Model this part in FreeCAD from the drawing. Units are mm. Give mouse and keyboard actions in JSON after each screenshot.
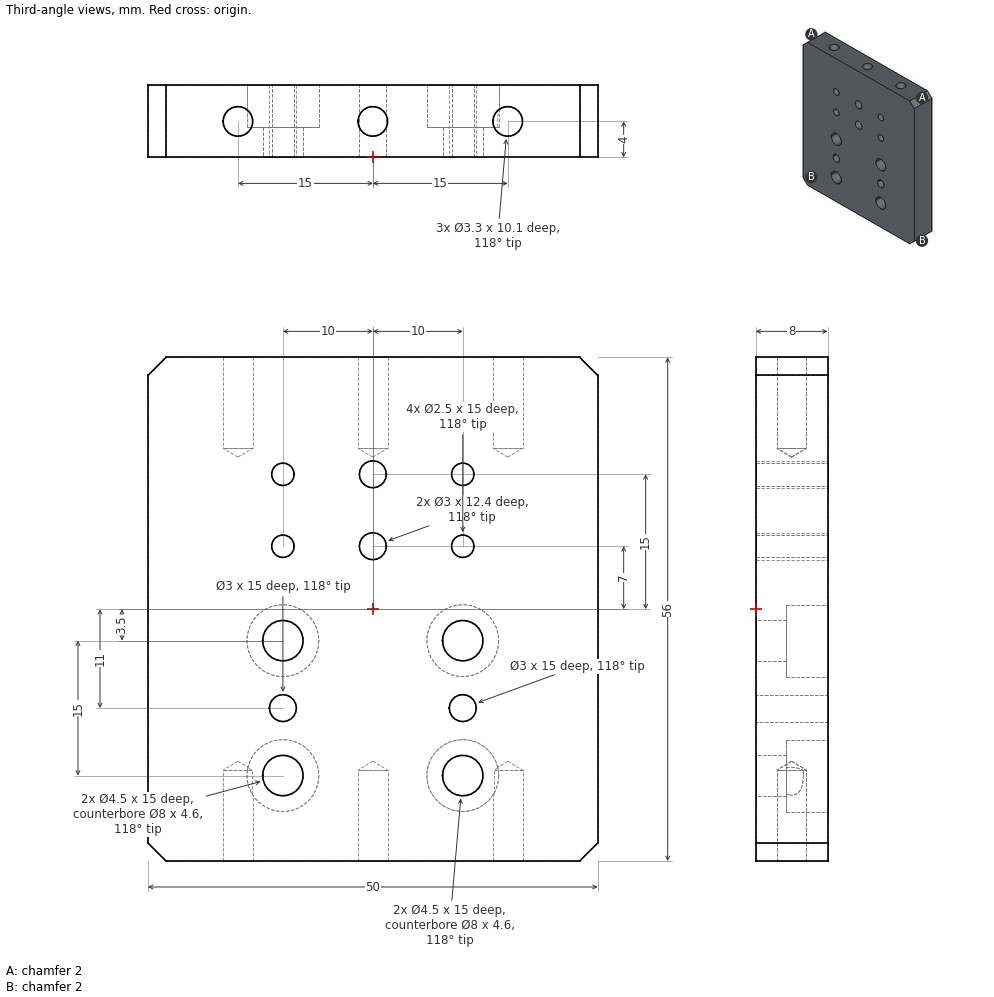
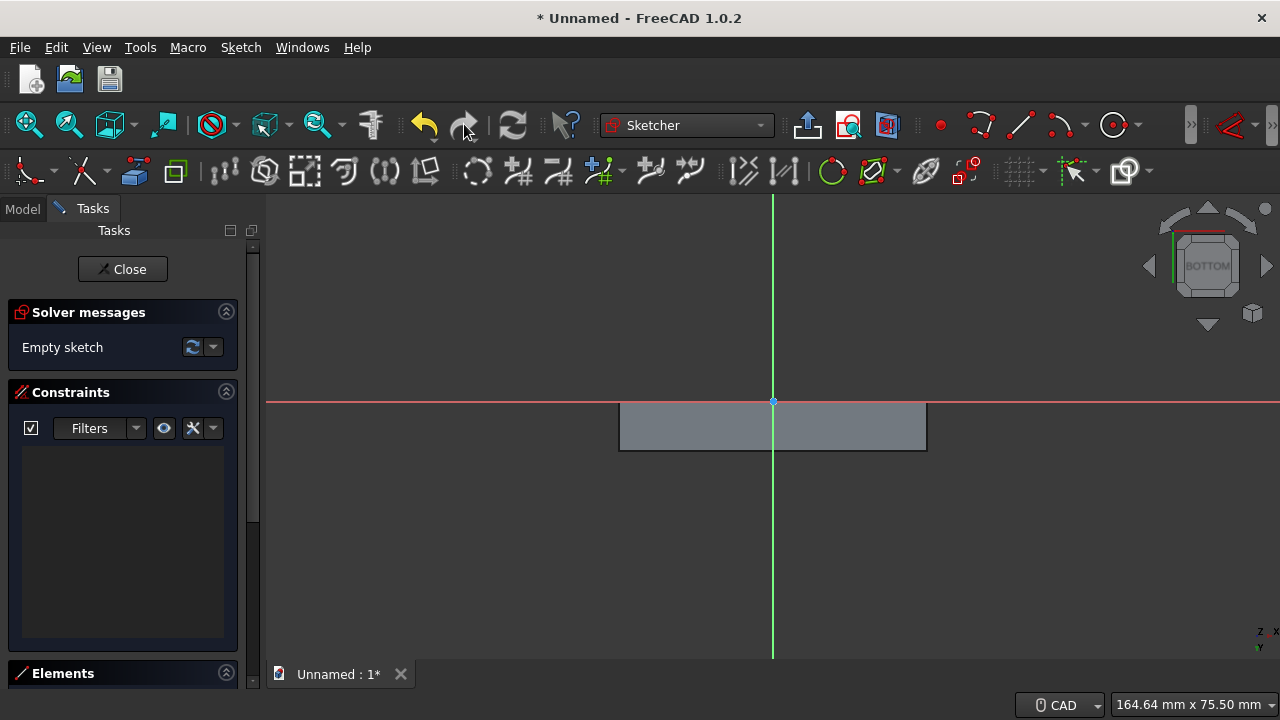
{"action": "scroll", "coordinate": [813, 415], "scroll_direction": "up", "scroll_amount": 5}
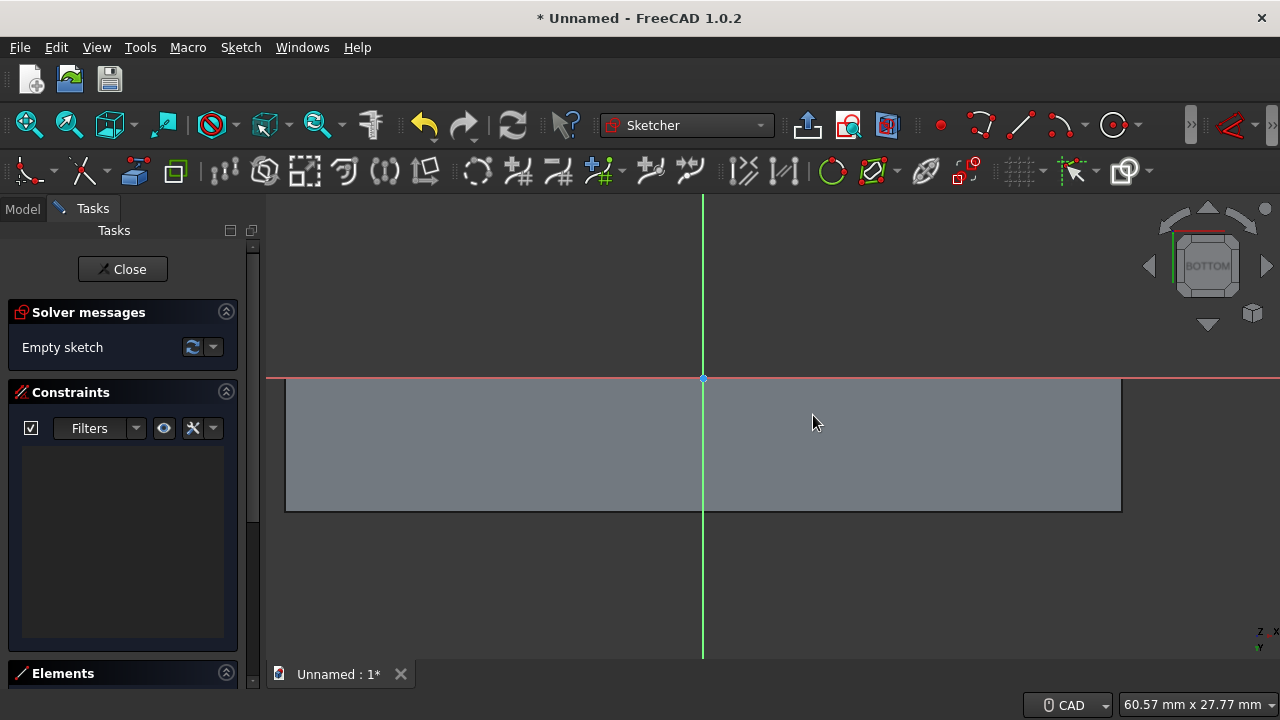
{"action": "left_click", "coordinate": [1114, 126]}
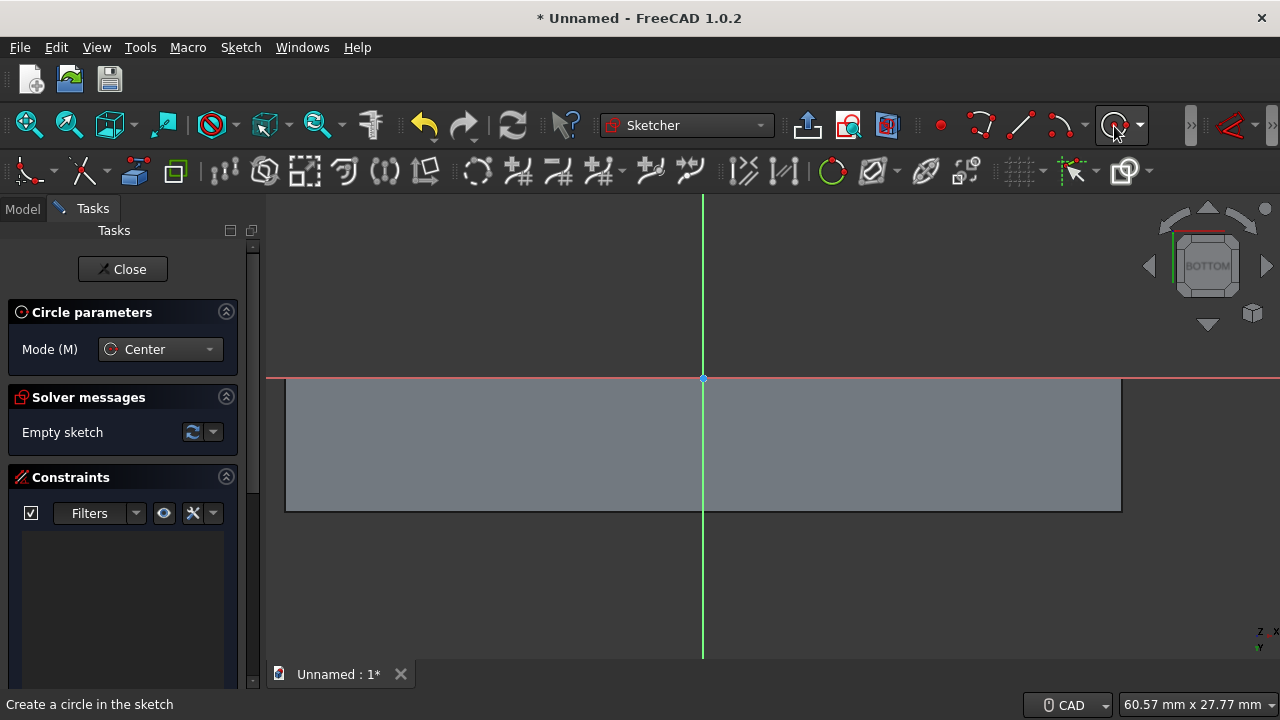
{"action": "left_click", "coordinate": [954, 445]}
{"action": "mouse_move", "coordinate": [974, 426]}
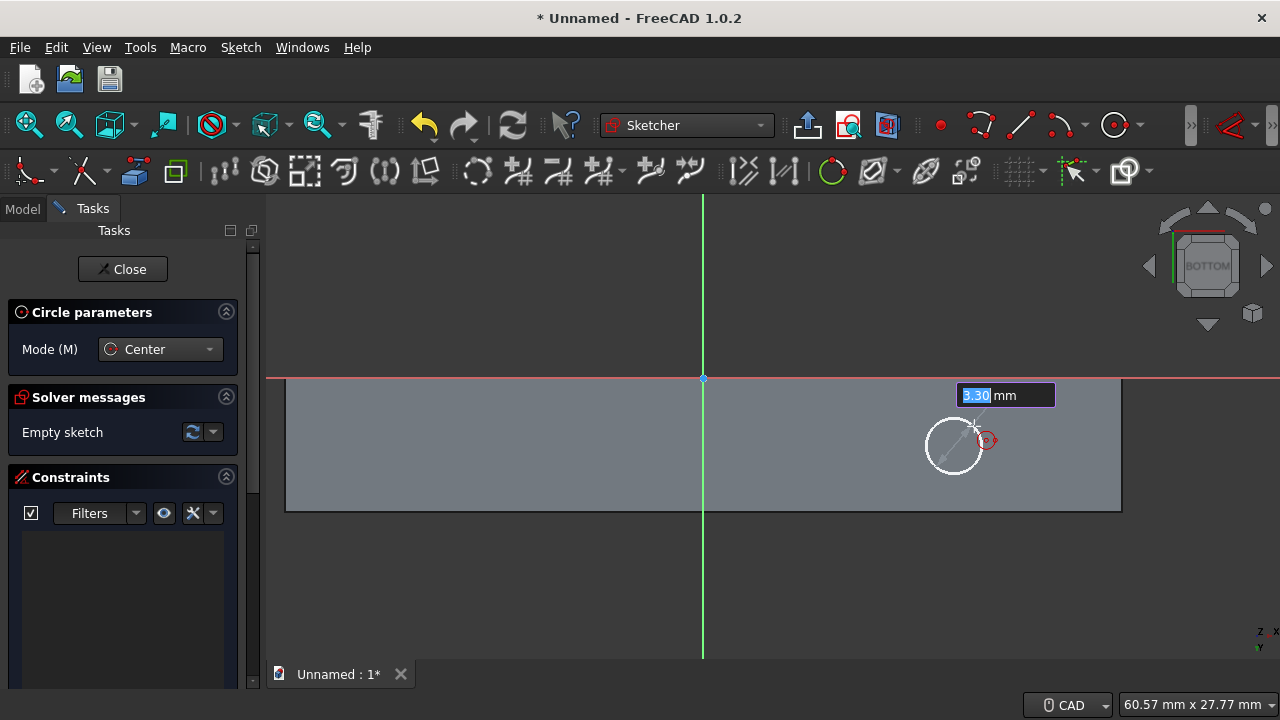
{"action": "type", "text": "3.3"}
{"action": "key", "text": "Return"}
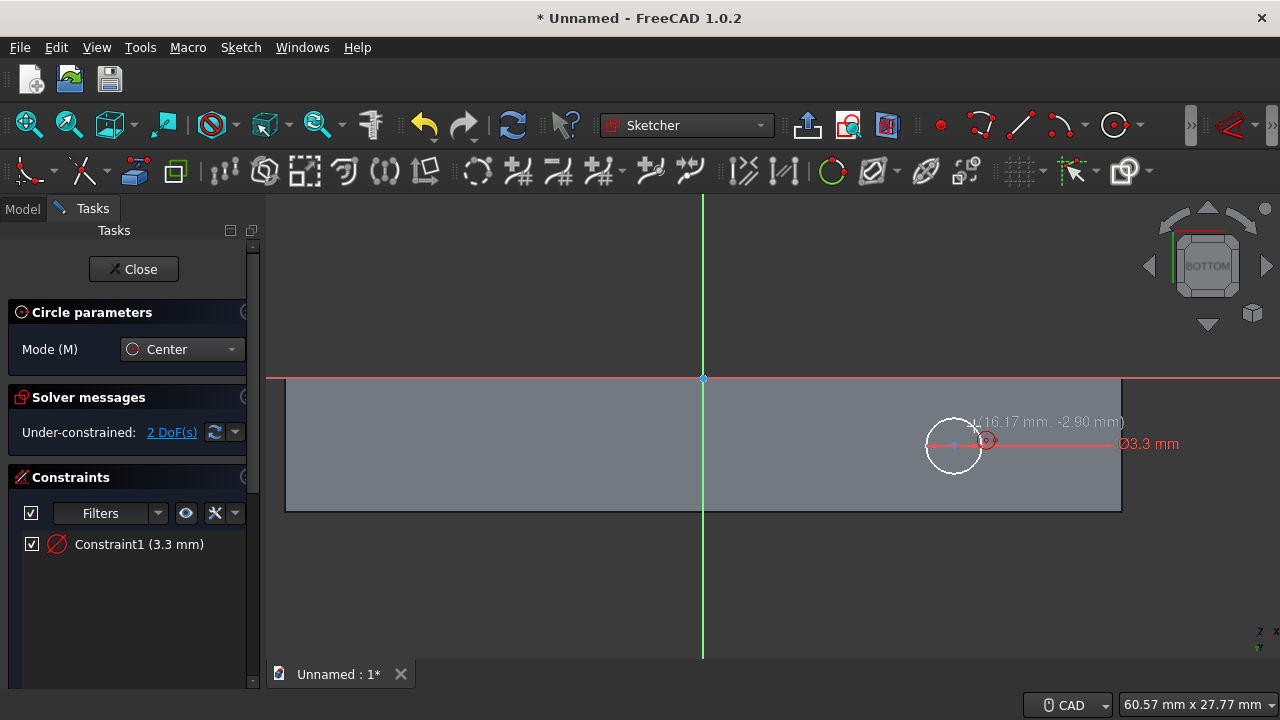
{"action": "left_click", "coordinate": [703, 445]}
{"action": "mouse_move", "coordinate": [723, 426]}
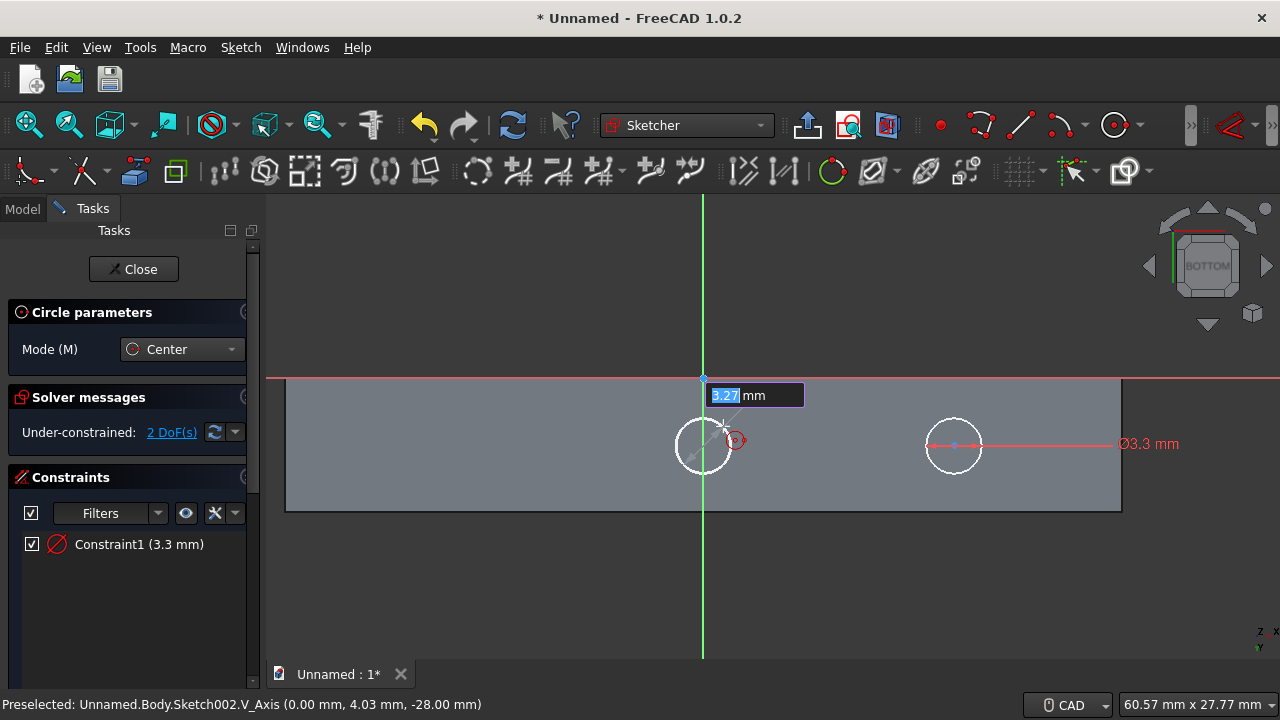
{"action": "type", "text": "3.3"}
{"action": "key", "text": "Return"}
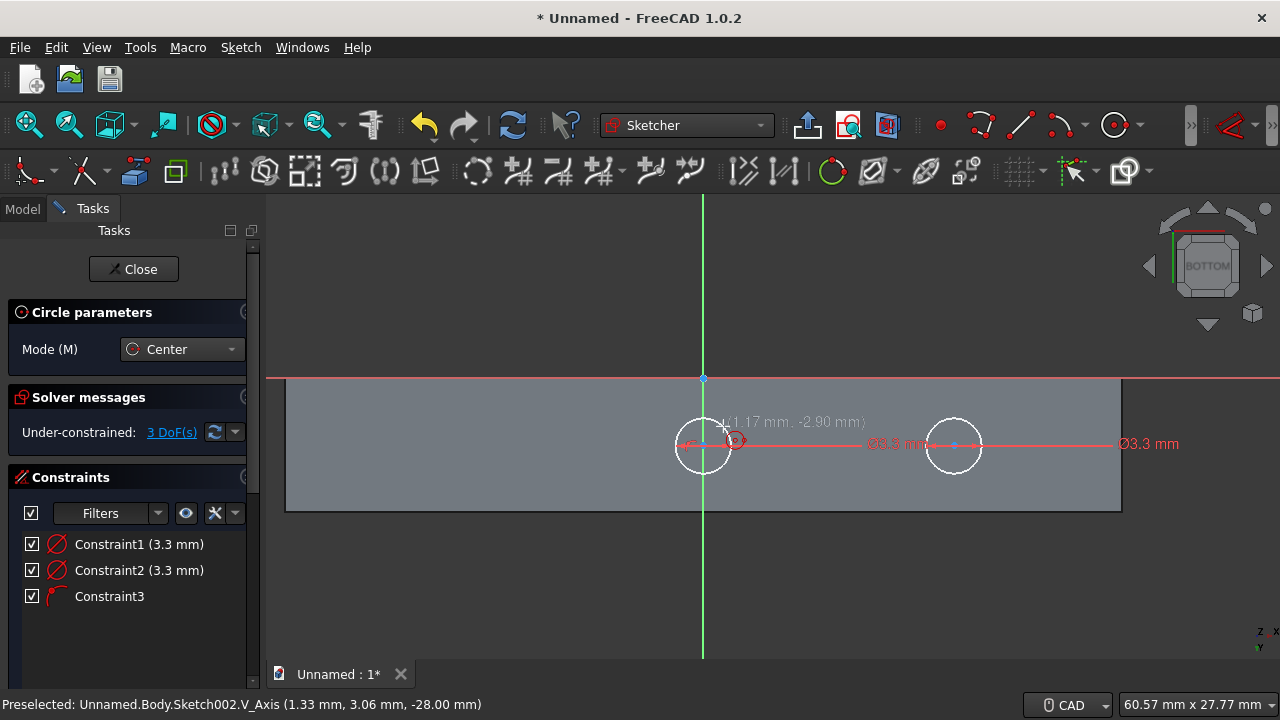
{"action": "left_click", "coordinate": [452, 445]}
{"action": "mouse_move", "coordinate": [472, 426]}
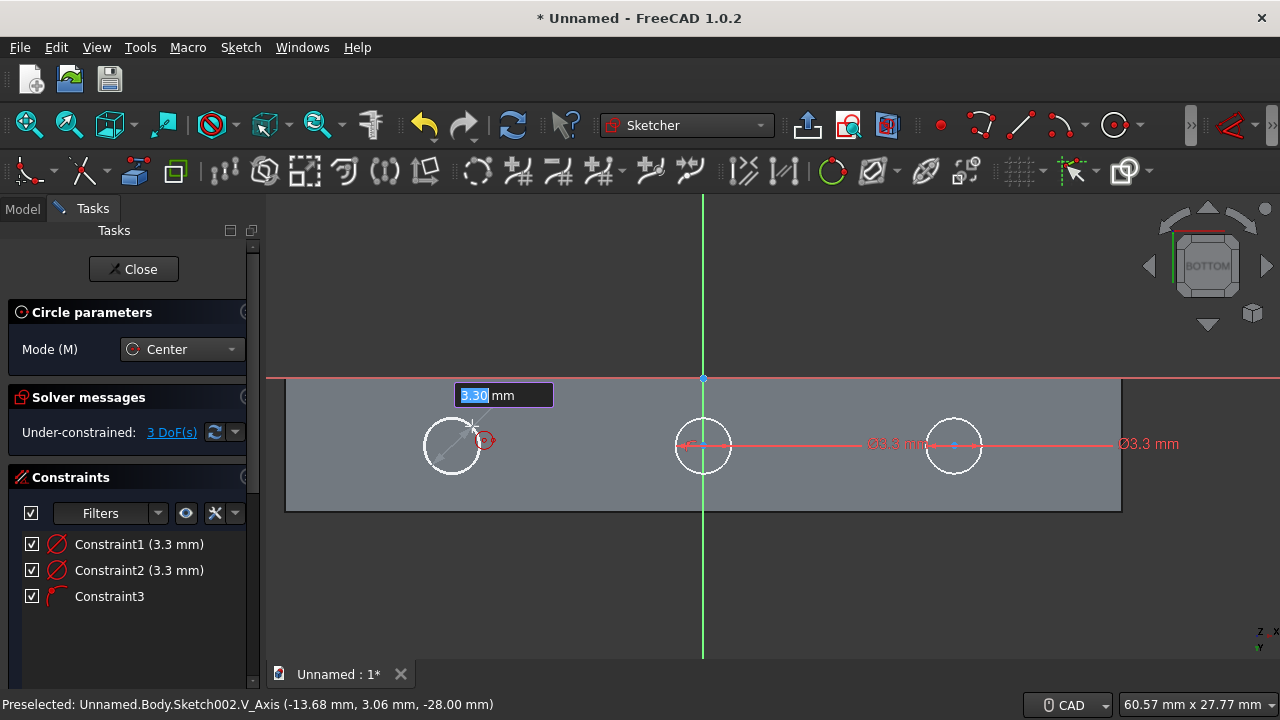
{"action": "type", "text": "3.3"}
{"action": "key", "text": "Return"}
{"action": "key", "text": "Escape"}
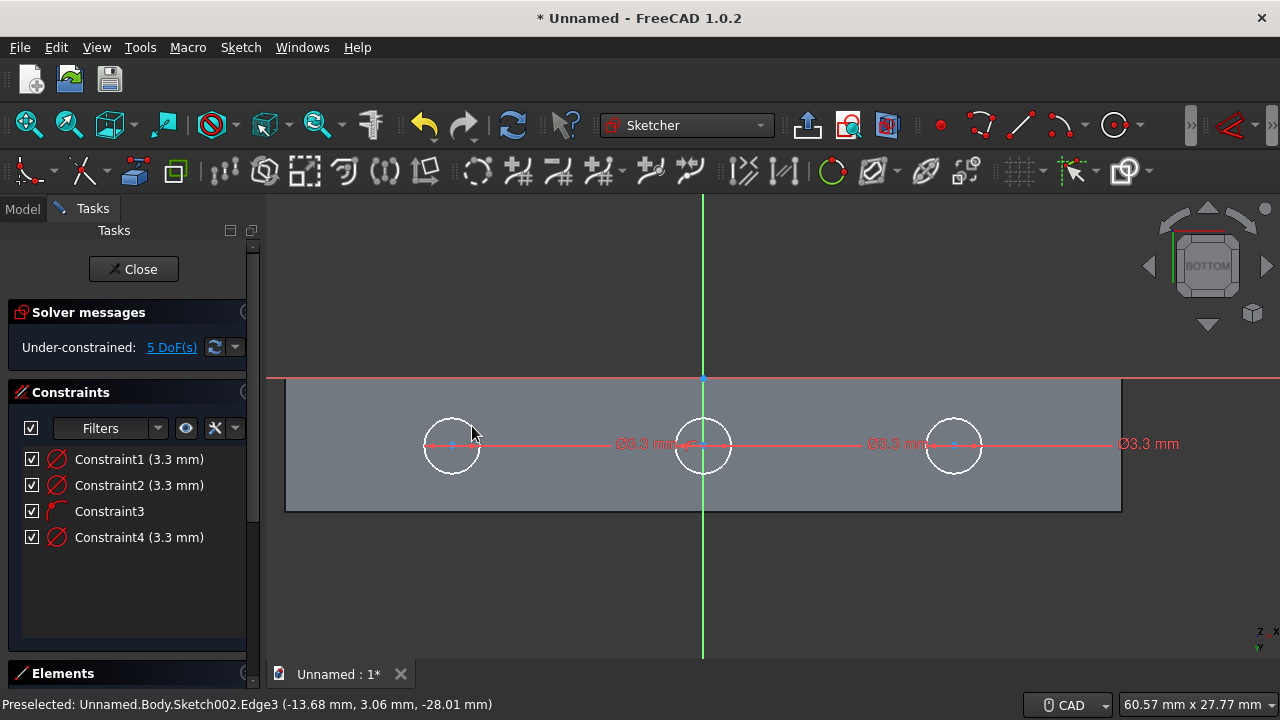
{"action": "left_click", "coordinate": [954, 446]}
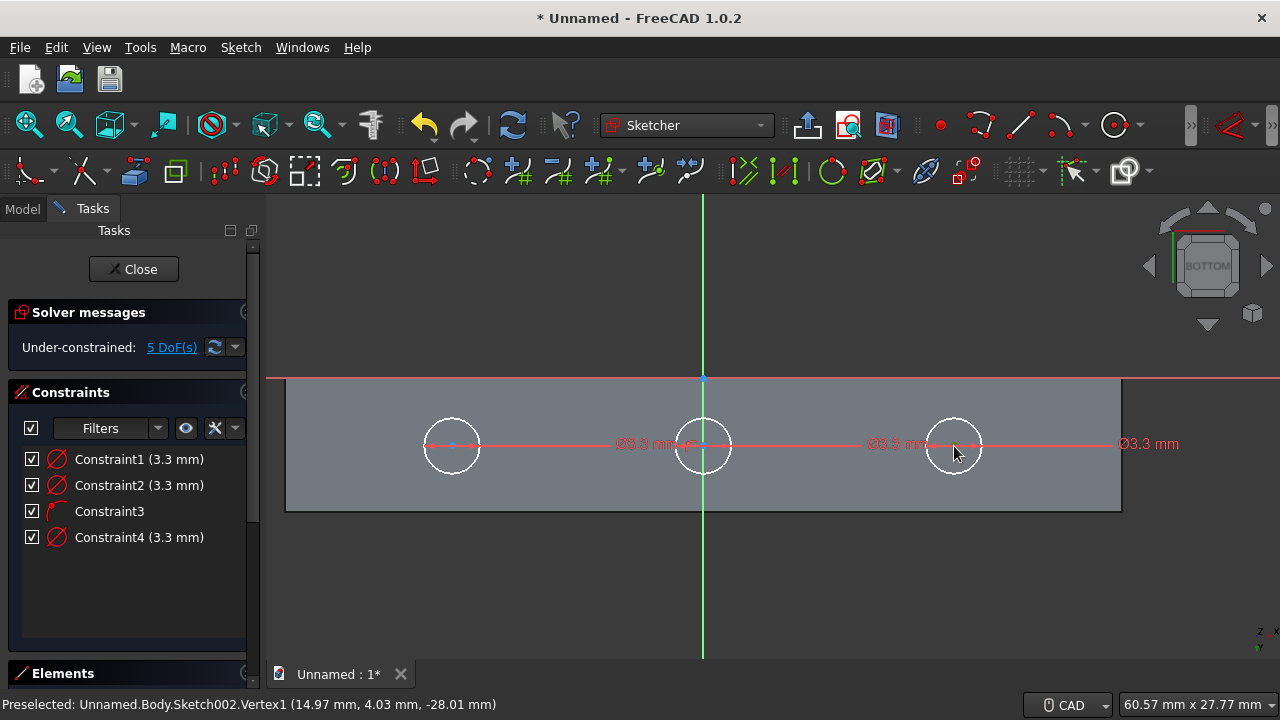
{"action": "left_click", "coordinate": [703, 446]}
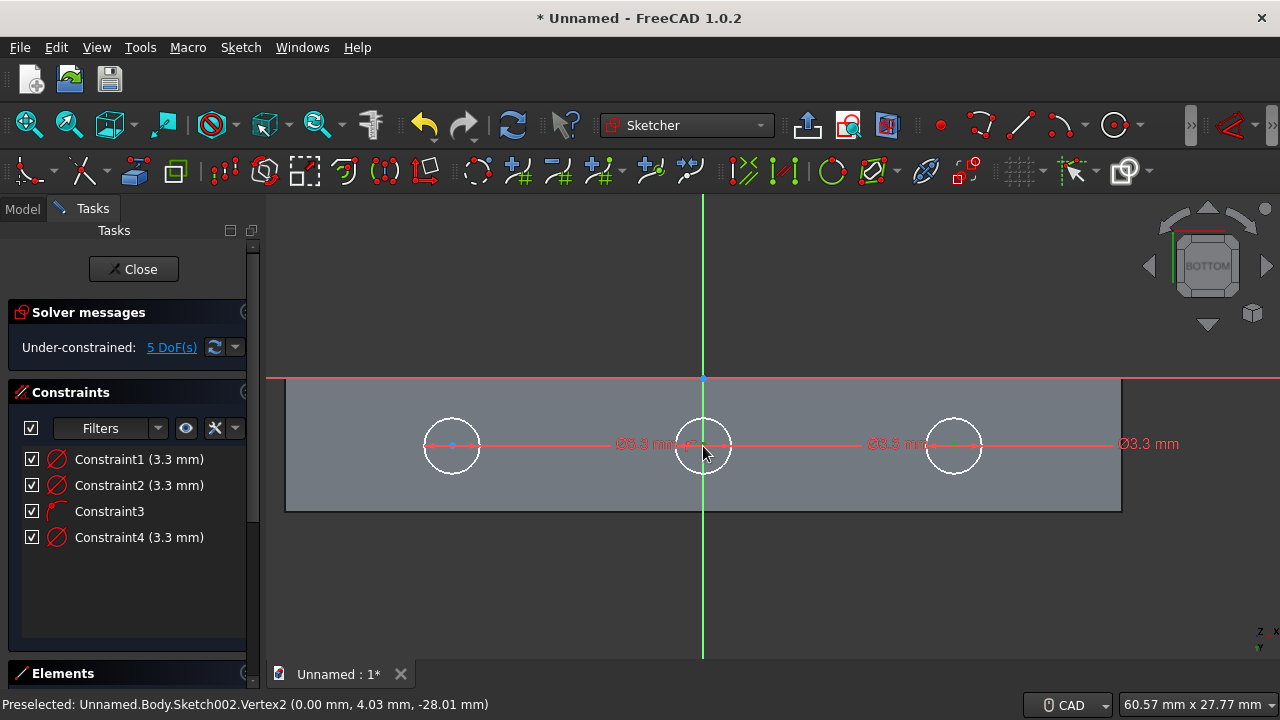
{"action": "key", "text": "h"}